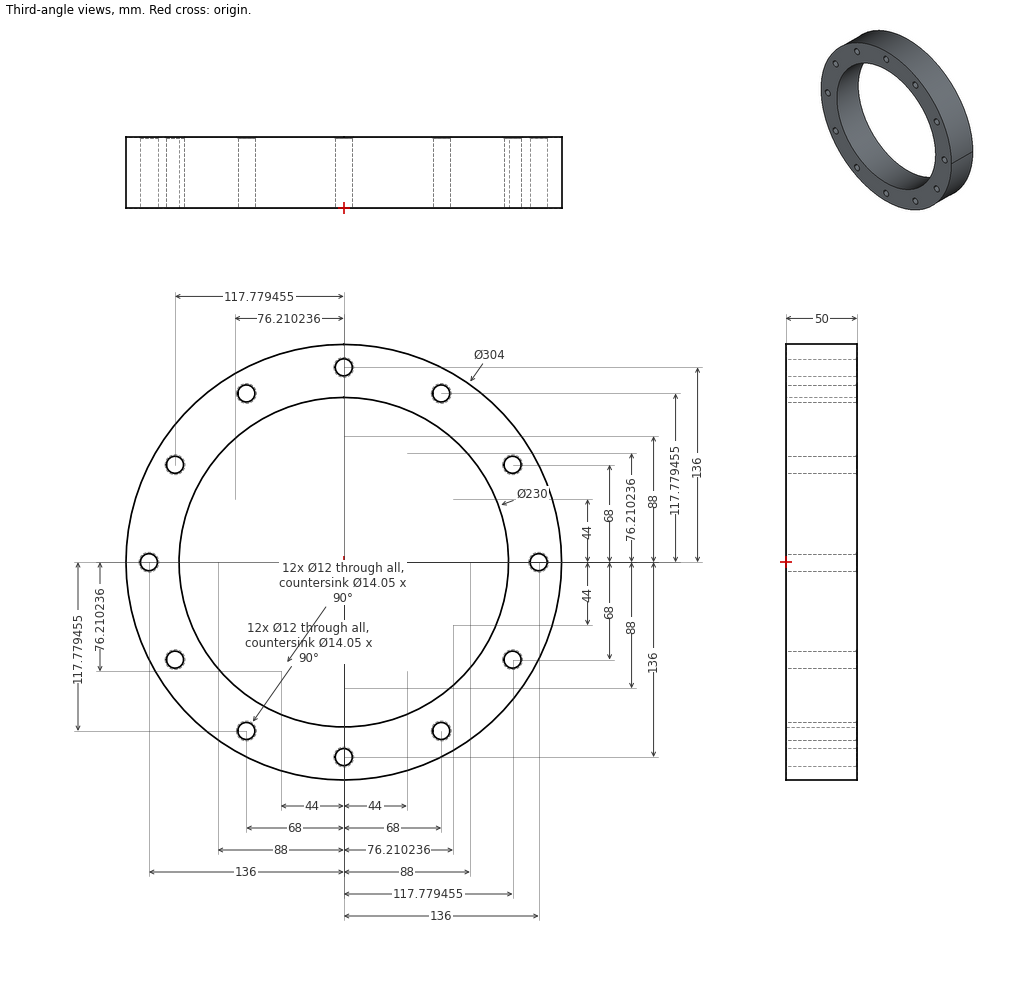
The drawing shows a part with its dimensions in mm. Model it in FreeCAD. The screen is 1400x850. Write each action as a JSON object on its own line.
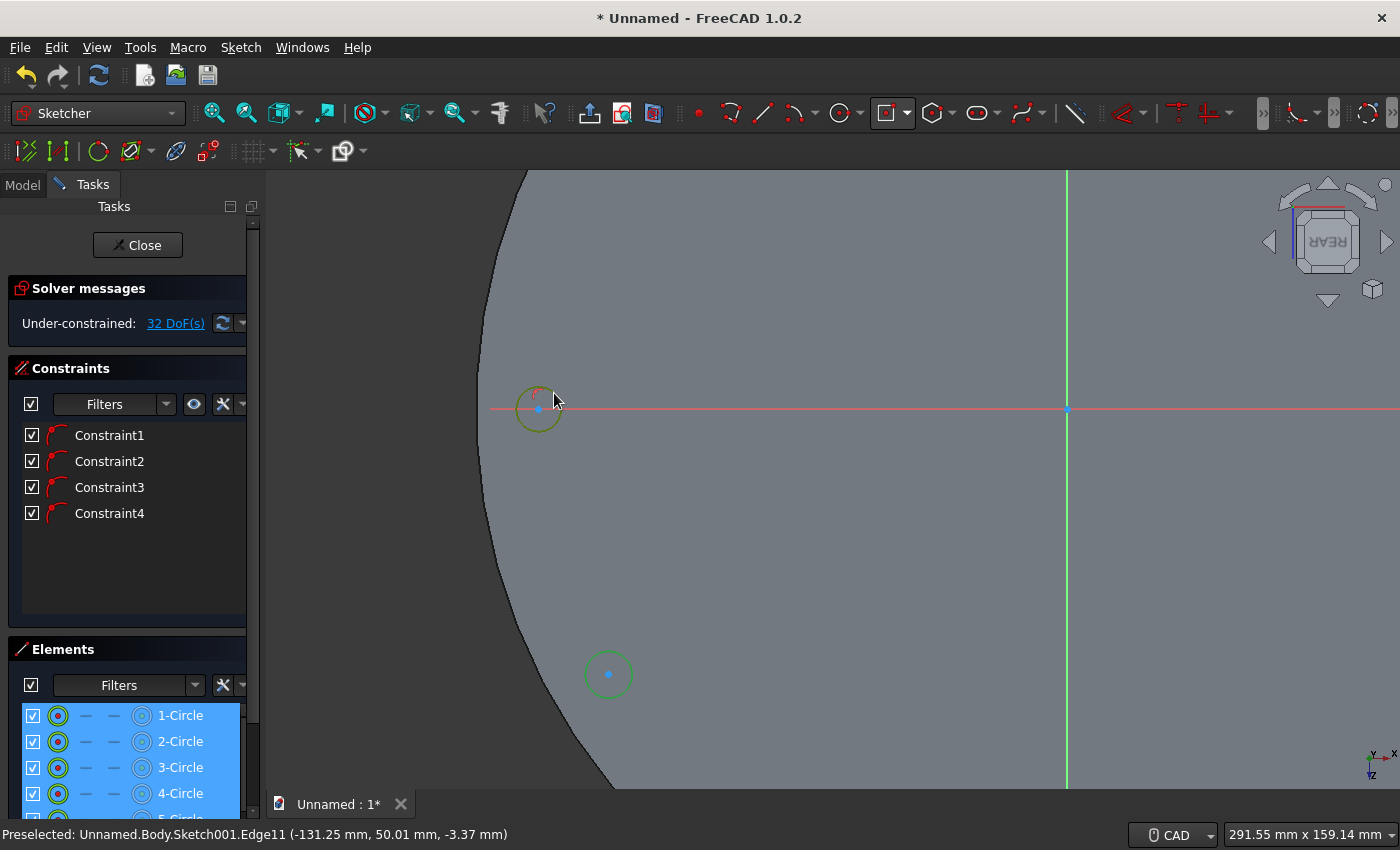
{"action": "scroll", "coordinate": [588, 520], "scroll_direction": "down", "scroll_amount": 5}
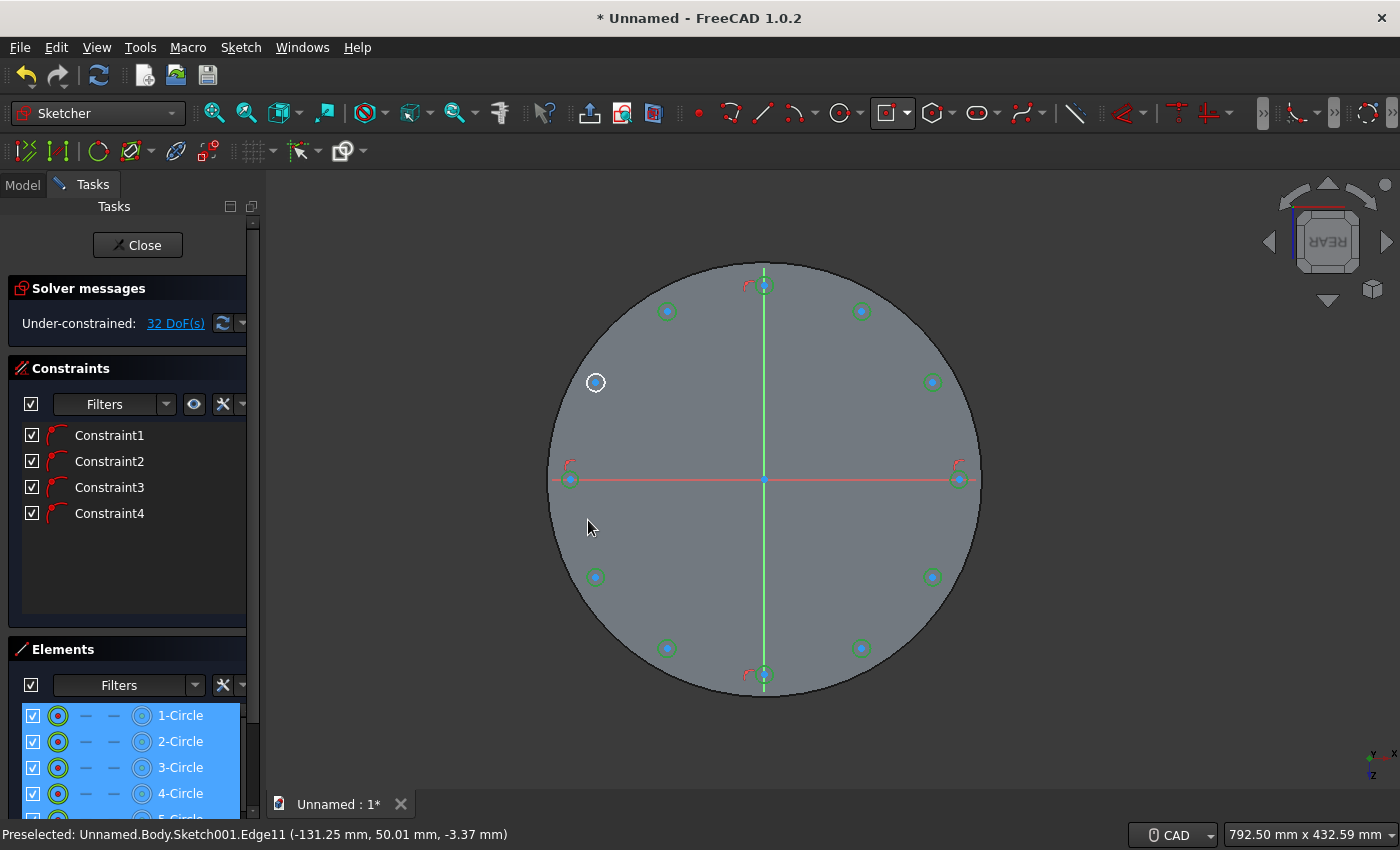
{"action": "scroll", "coordinate": [602, 376], "scroll_direction": "up", "scroll_amount": 3}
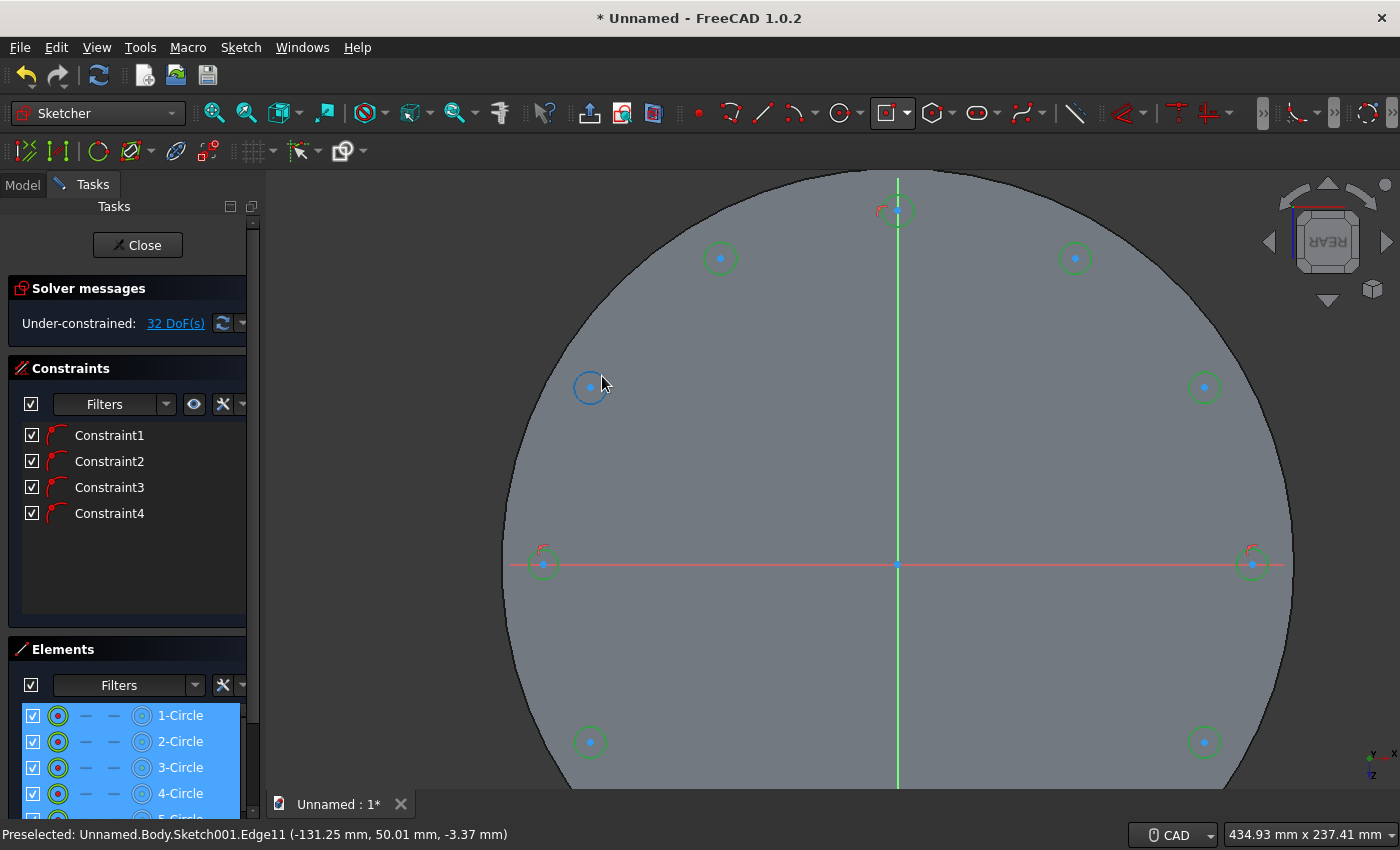
{"action": "left_click", "coordinate": [602, 377]}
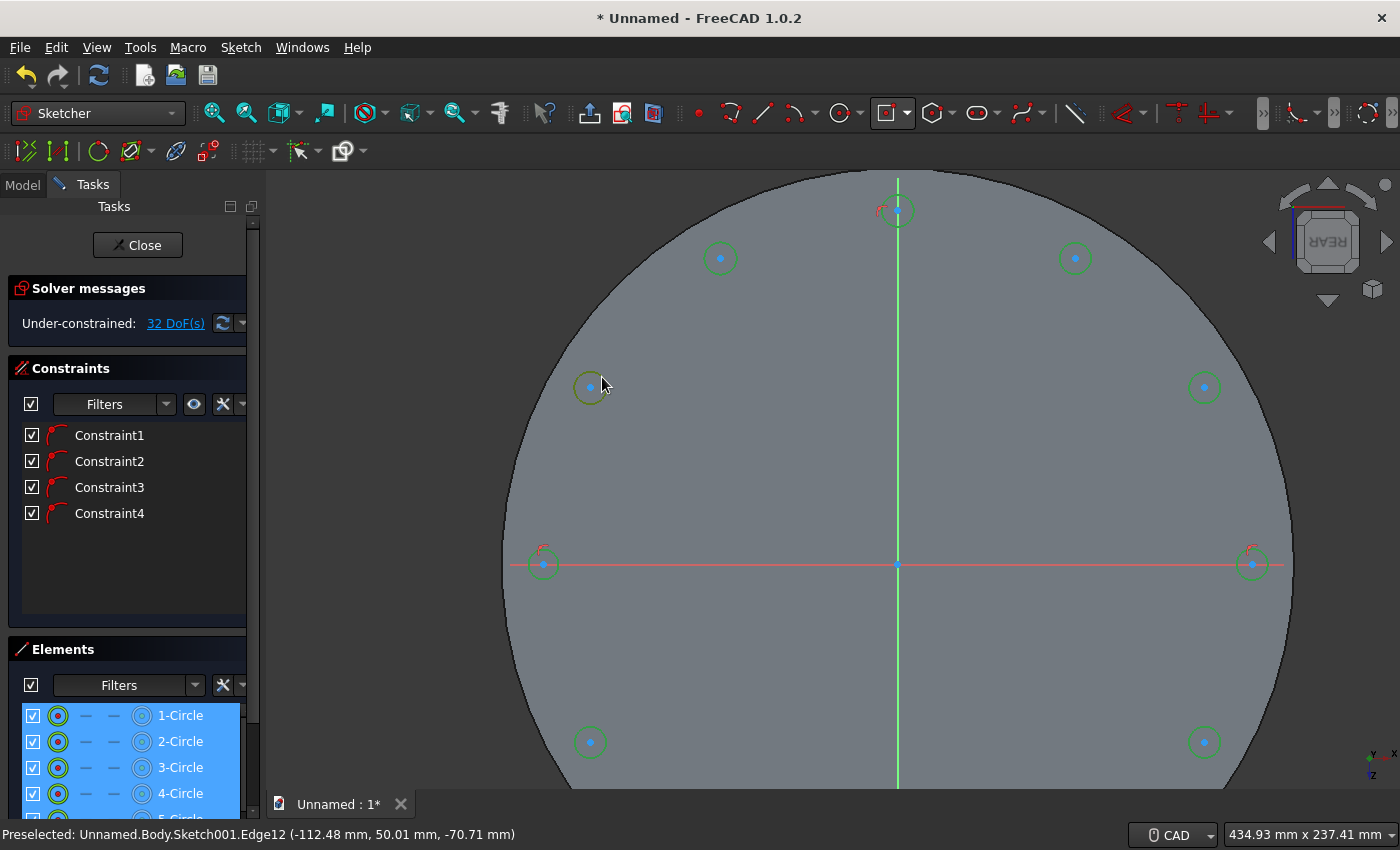
{"action": "key", "text": "e"}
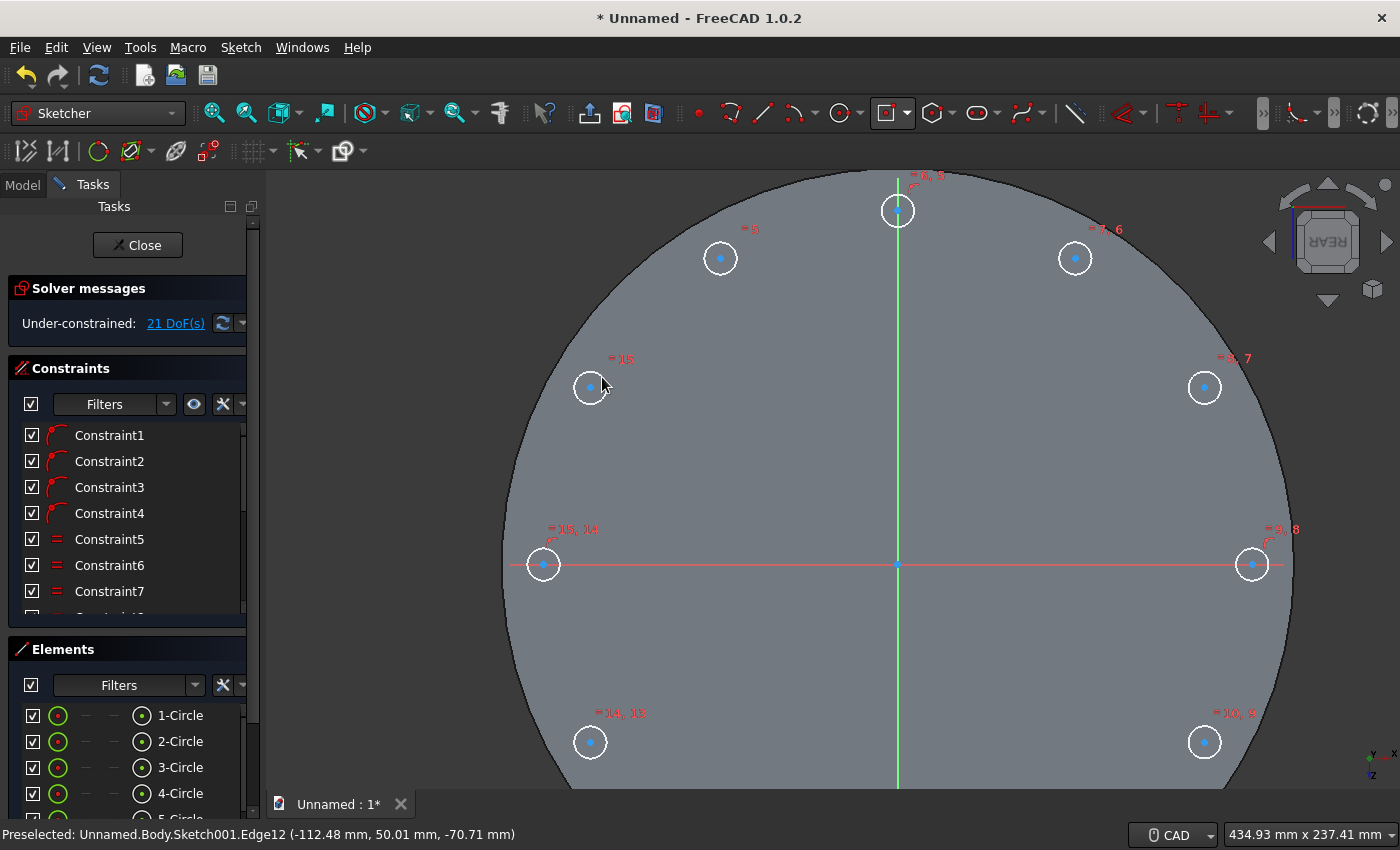
{"action": "left_click", "coordinate": [721, 258]}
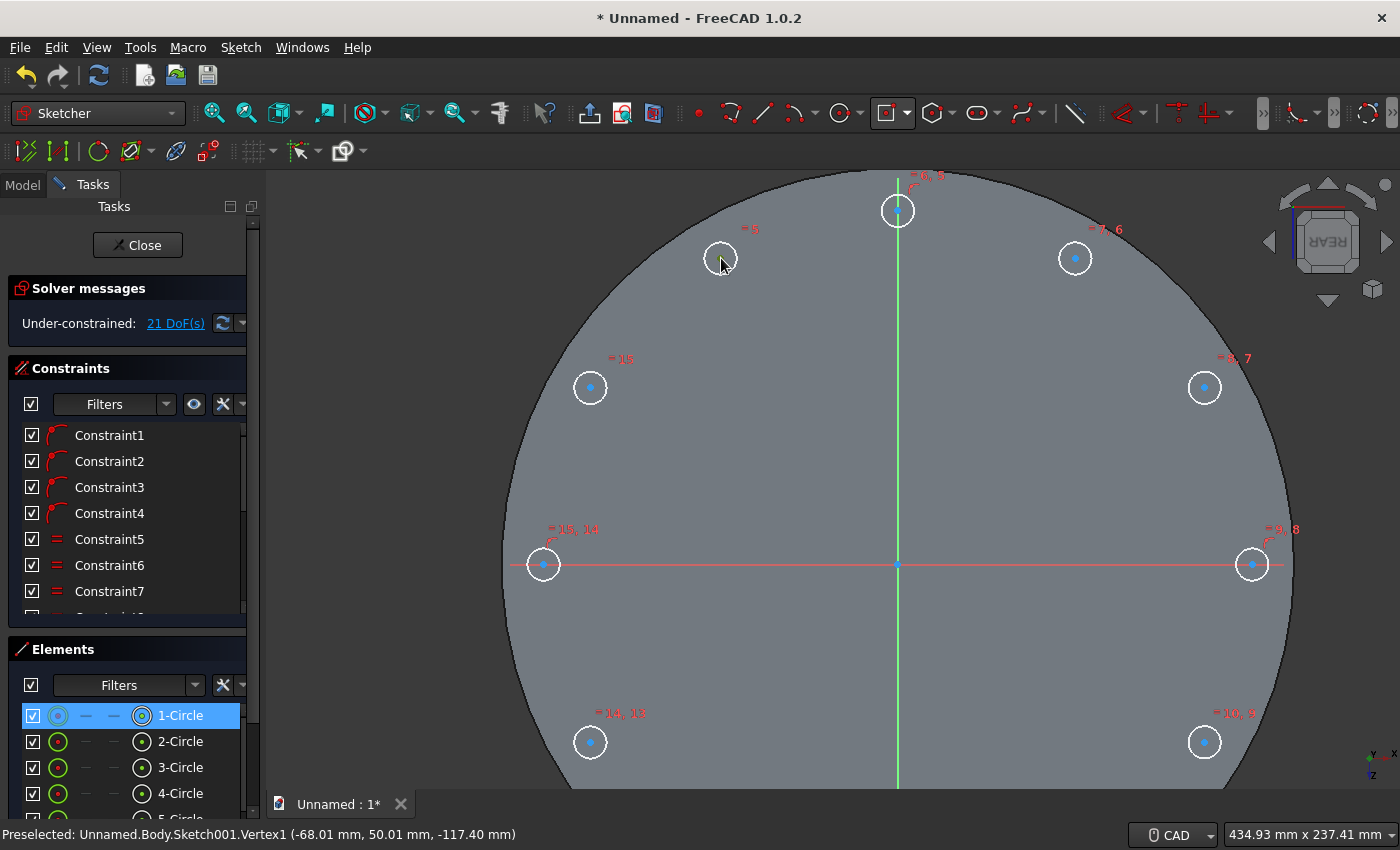
{"action": "left_click", "coordinate": [1075, 258]}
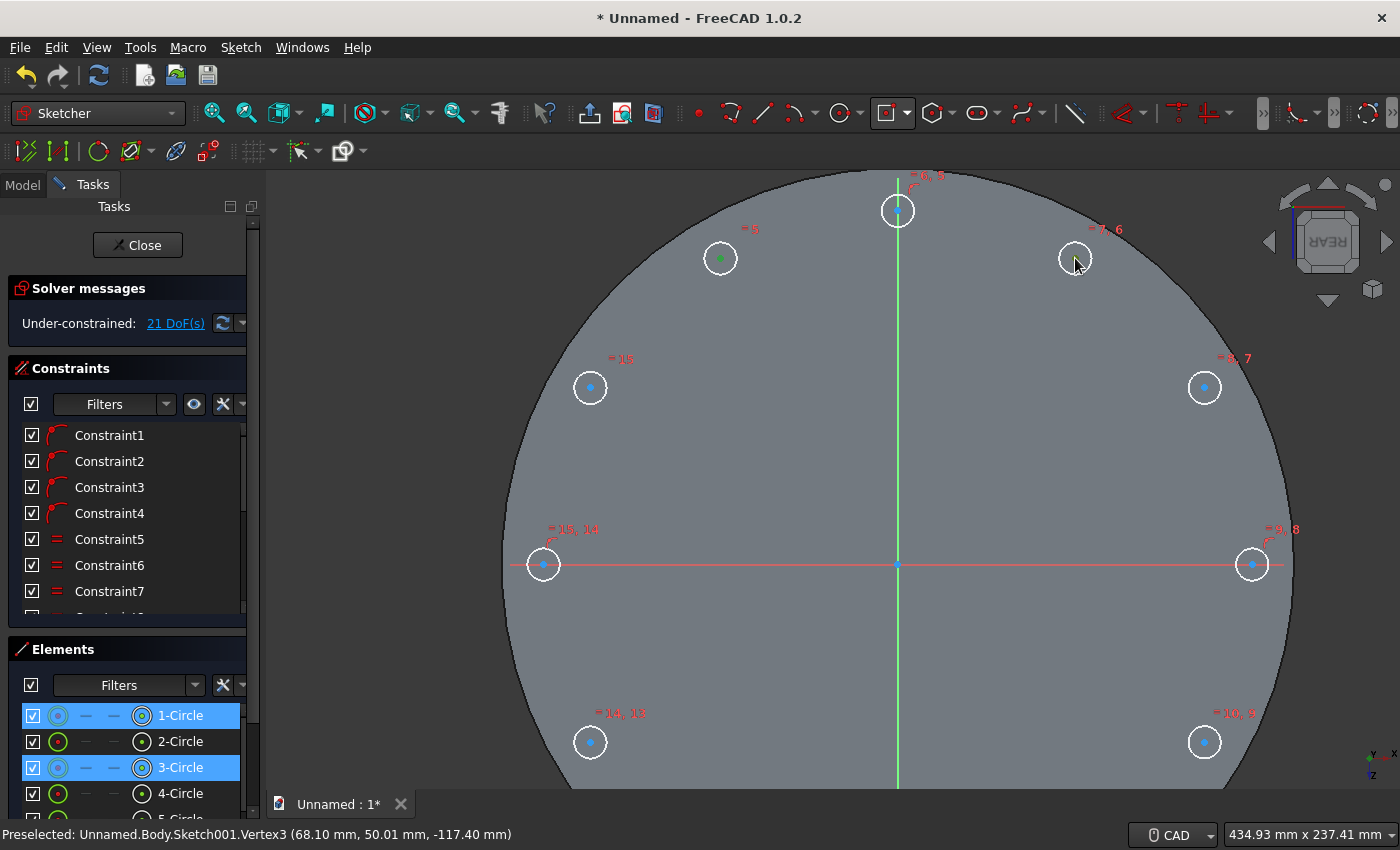
{"action": "key", "text": "h"}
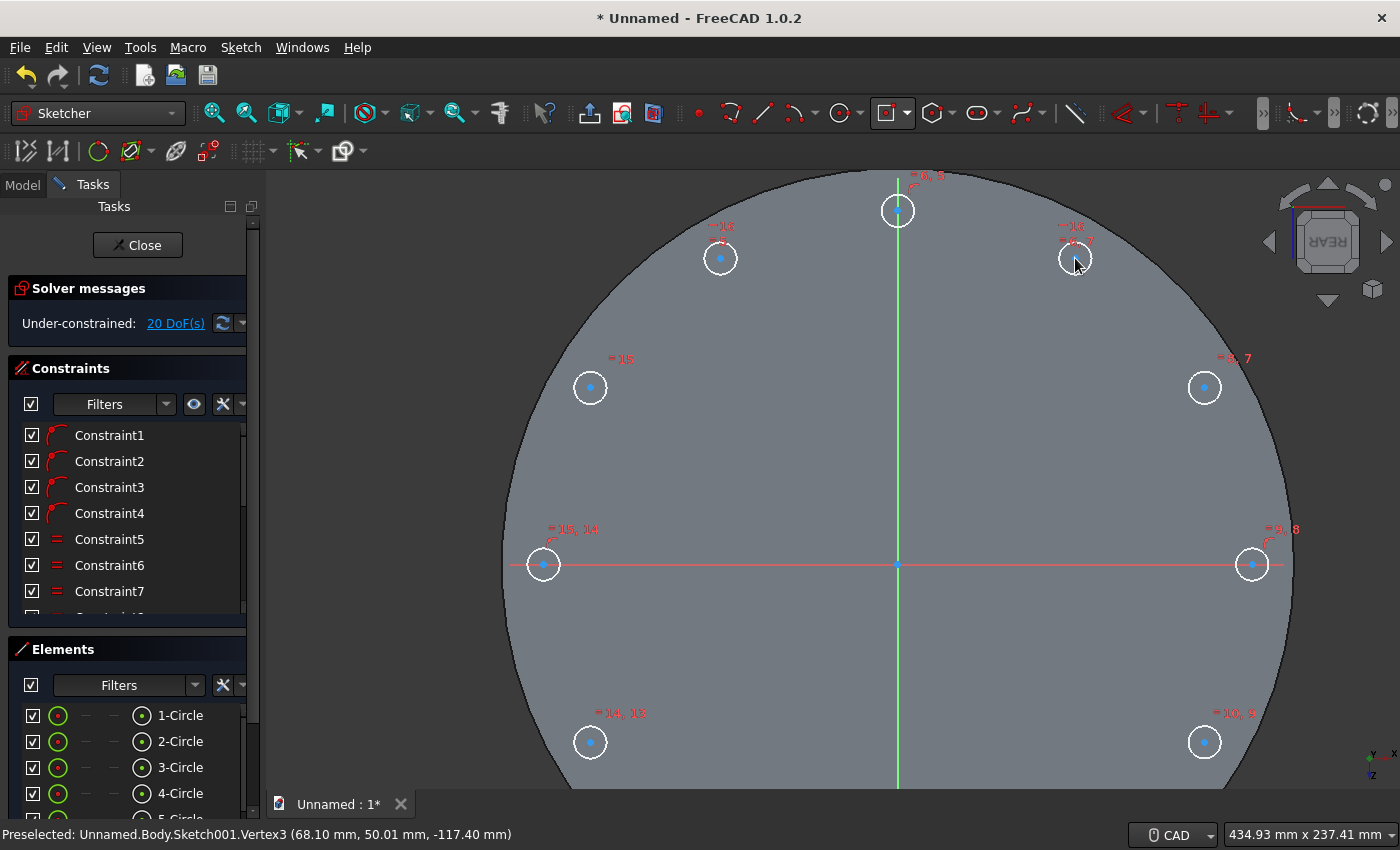
{"action": "left_click", "coordinate": [1205, 388]}